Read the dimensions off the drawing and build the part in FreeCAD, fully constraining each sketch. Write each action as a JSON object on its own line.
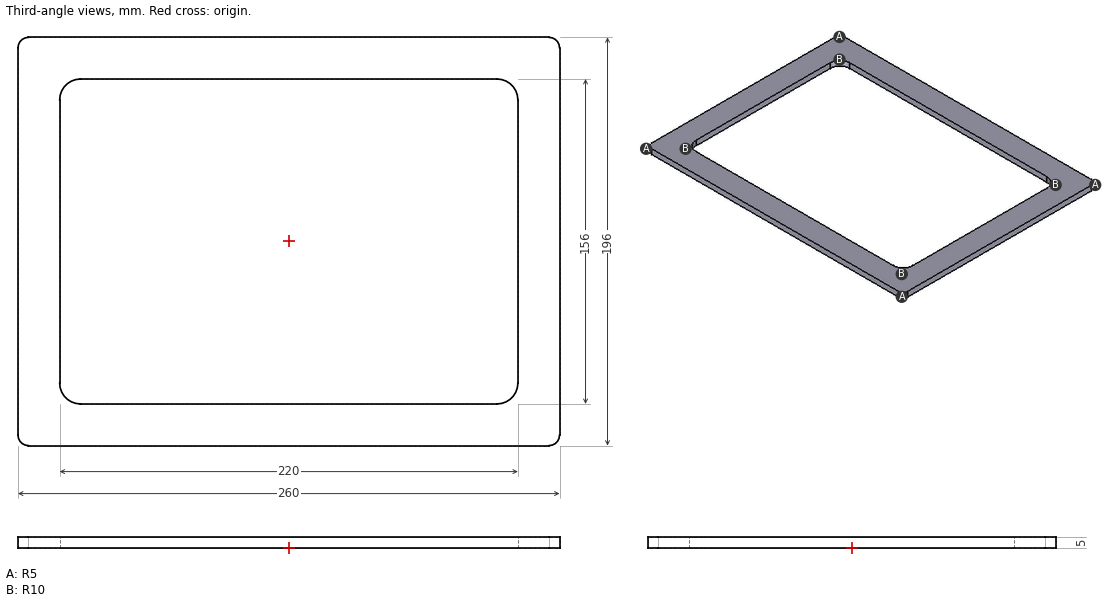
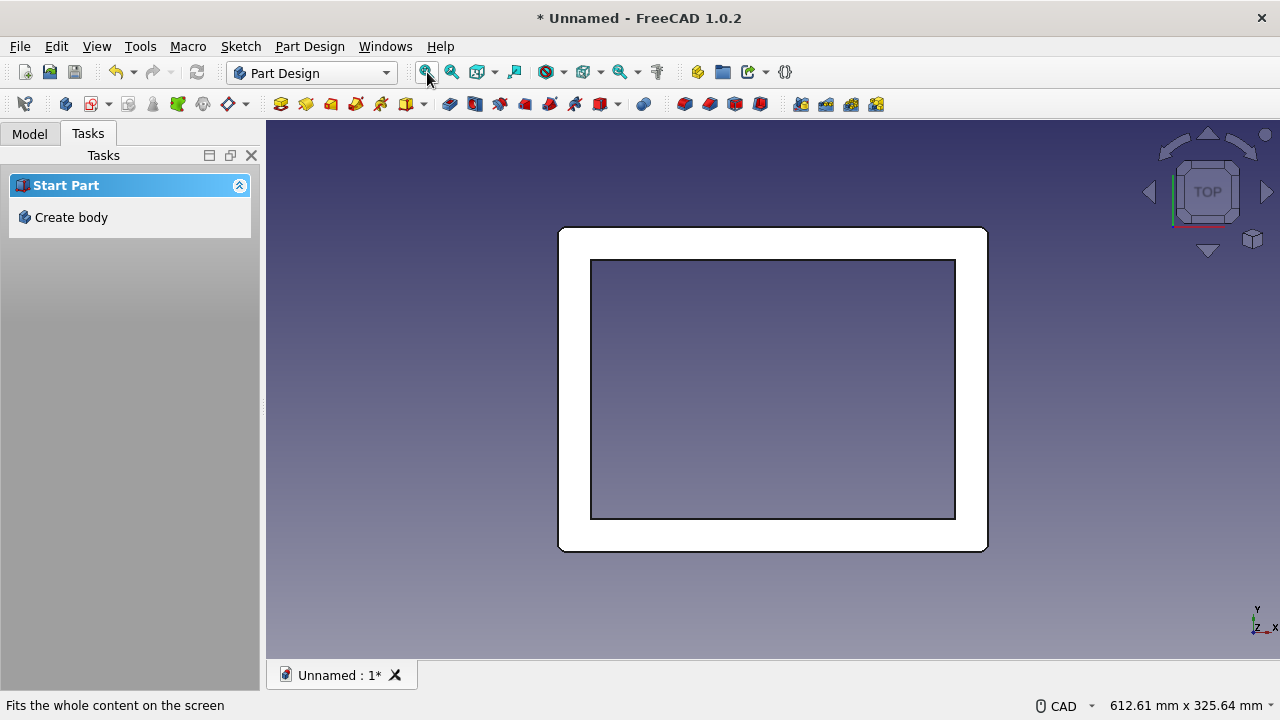
{"action": "key", "text": "0"}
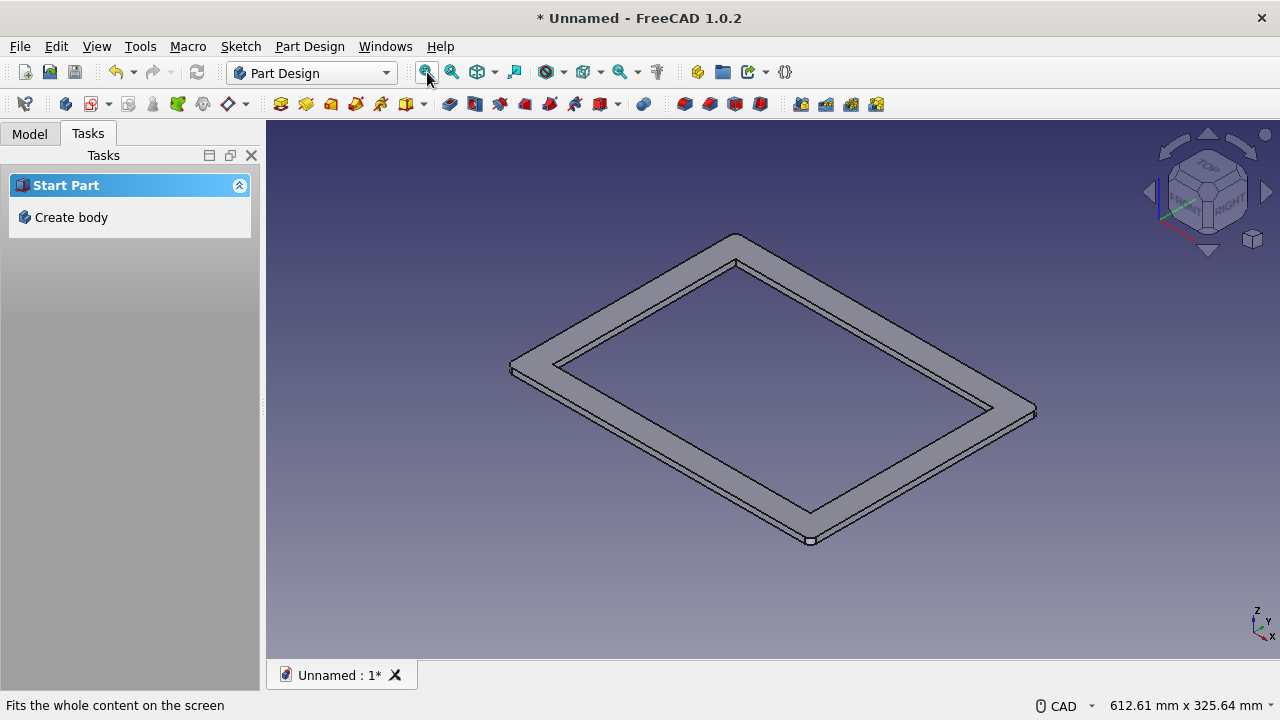
{"action": "scroll", "coordinate": [736, 261], "scroll_direction": "up", "scroll_amount": 8}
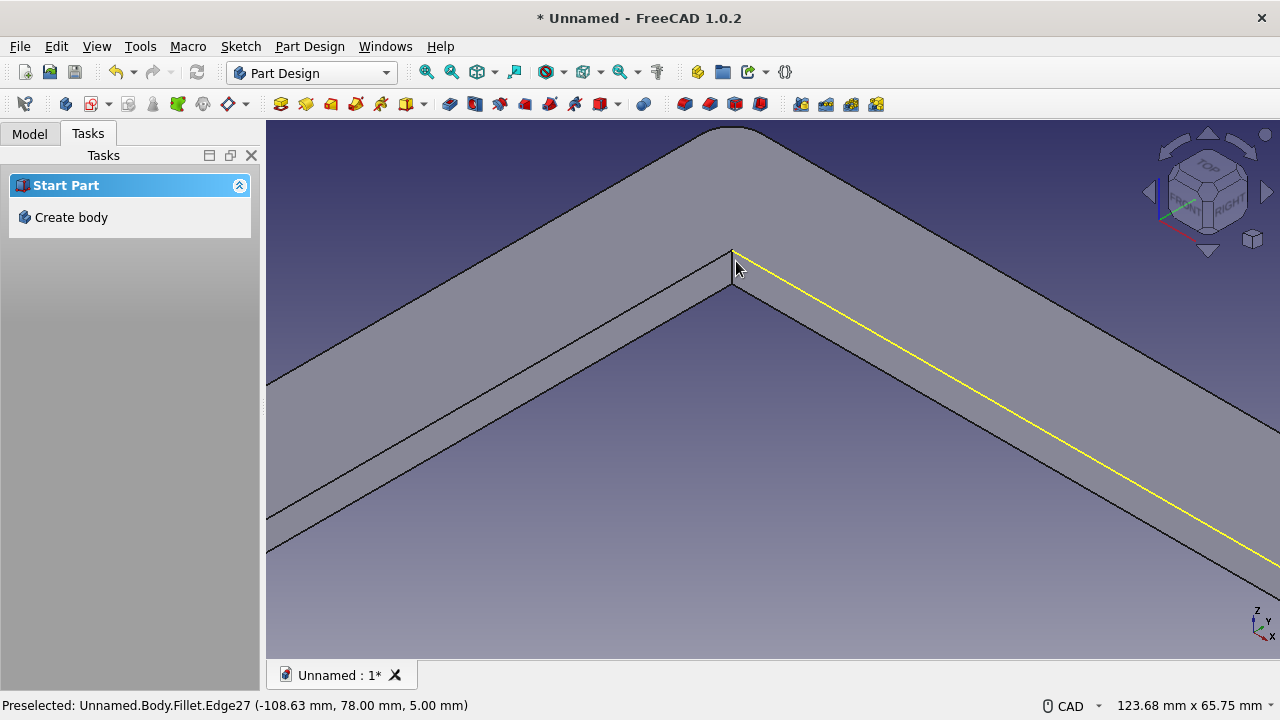
{"action": "left_click", "coordinate": [427, 72]}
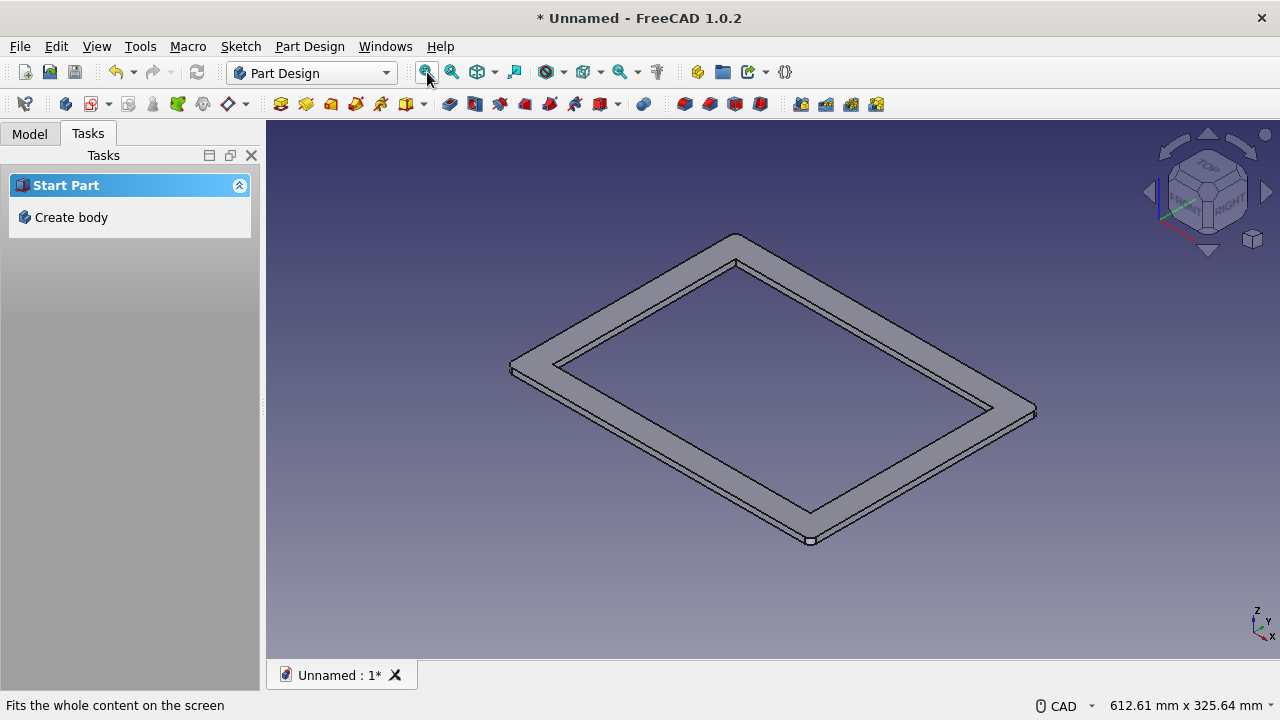
{"action": "key", "text": "1"}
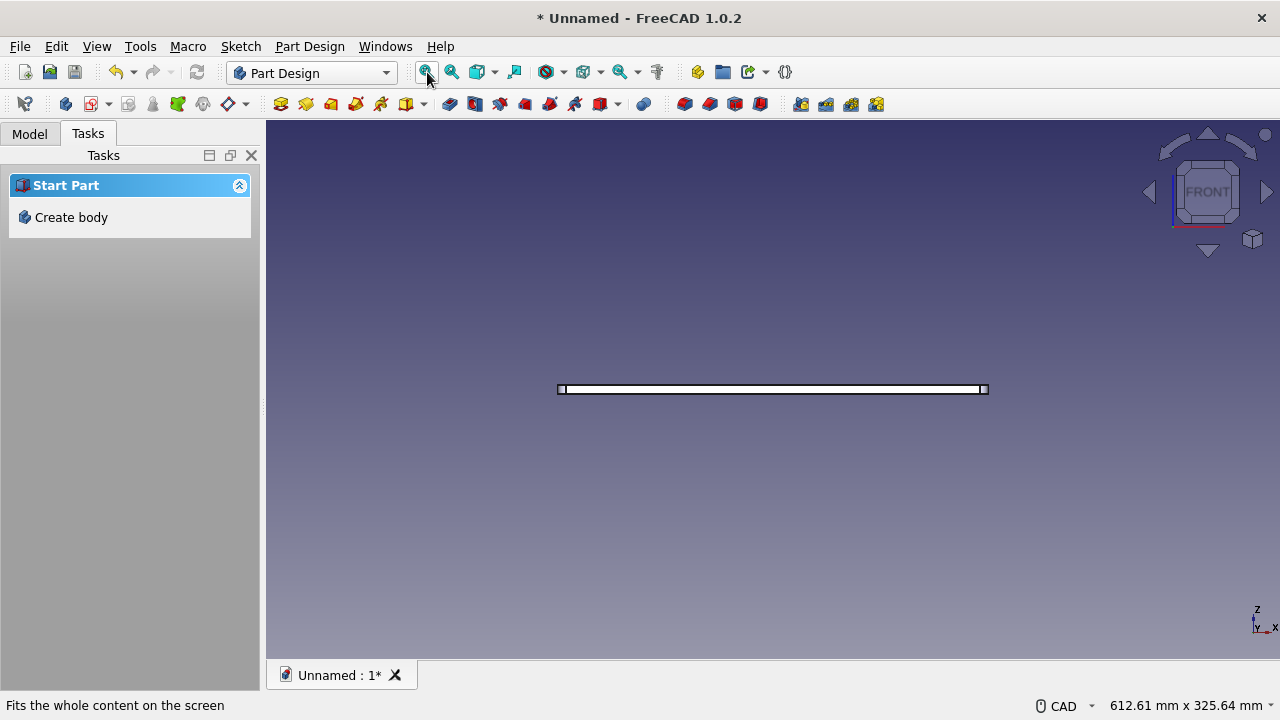
{"action": "left_click", "coordinate": [427, 72]}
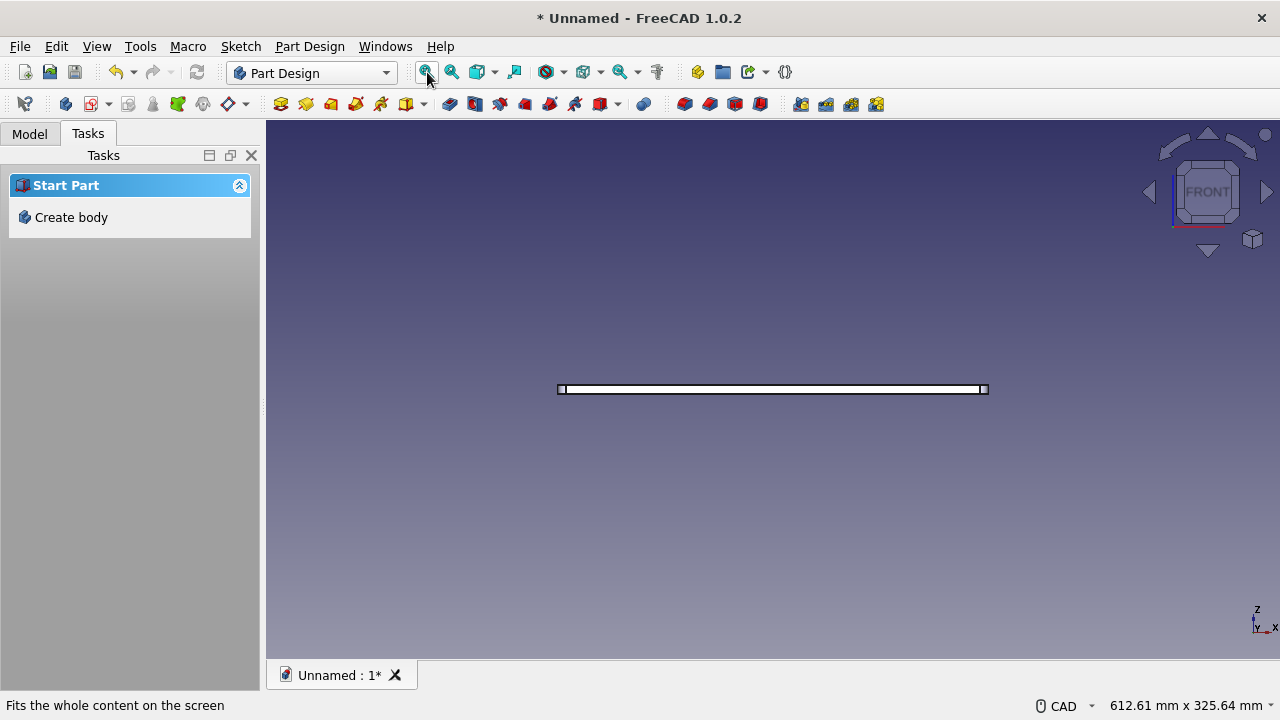
{"action": "scroll", "coordinate": [591, 389], "scroll_direction": "up", "scroll_amount": 8}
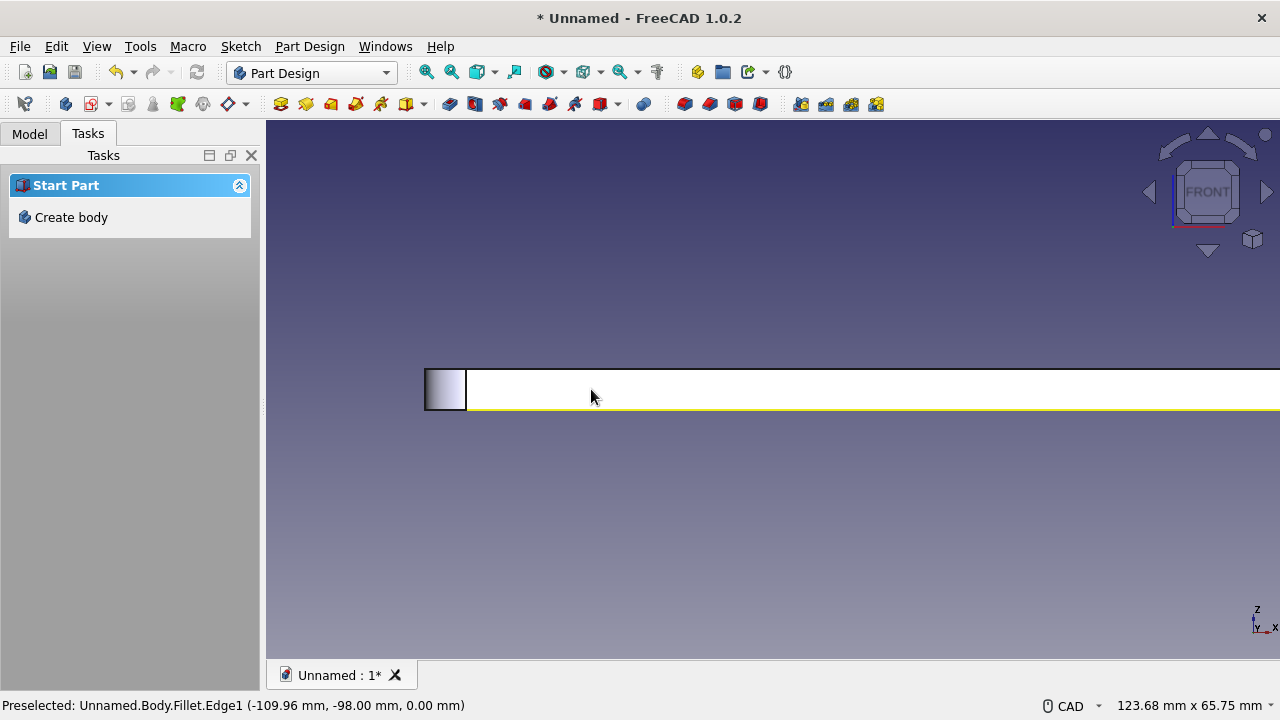
{"action": "left_click", "coordinate": [427, 72]}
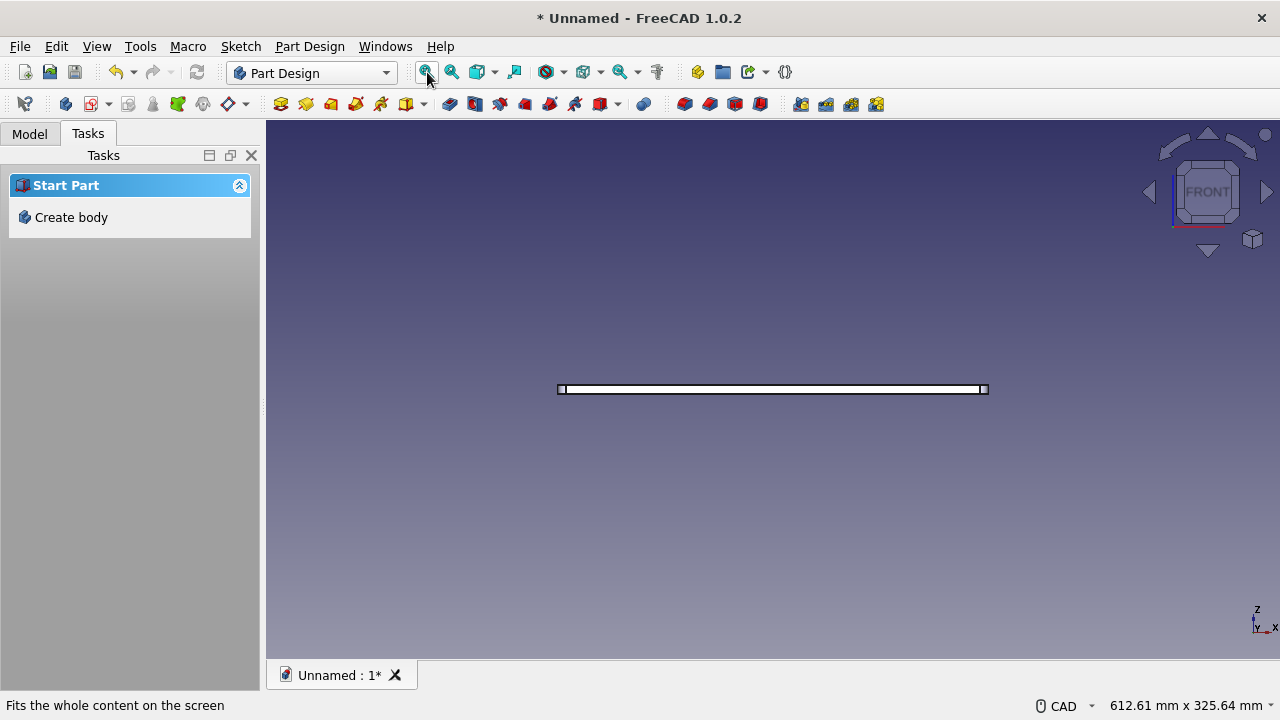
{"action": "key", "text": "3"}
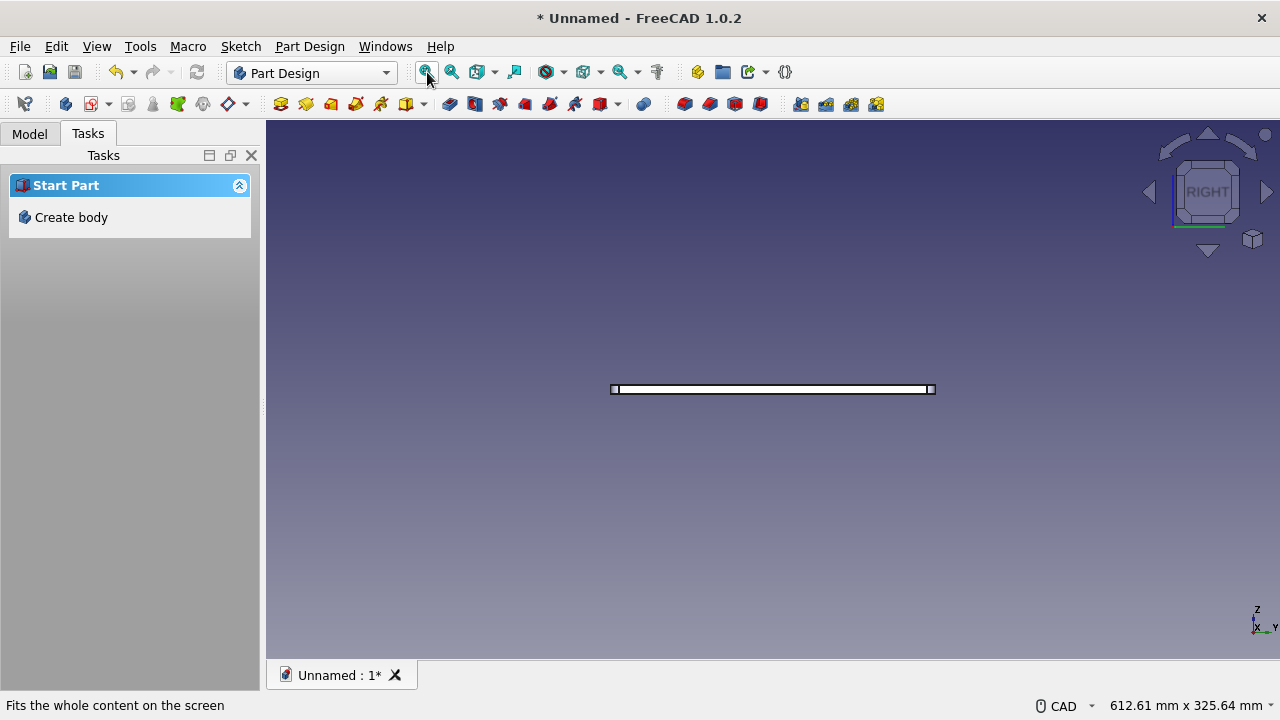
{"action": "left_click", "coordinate": [427, 72]}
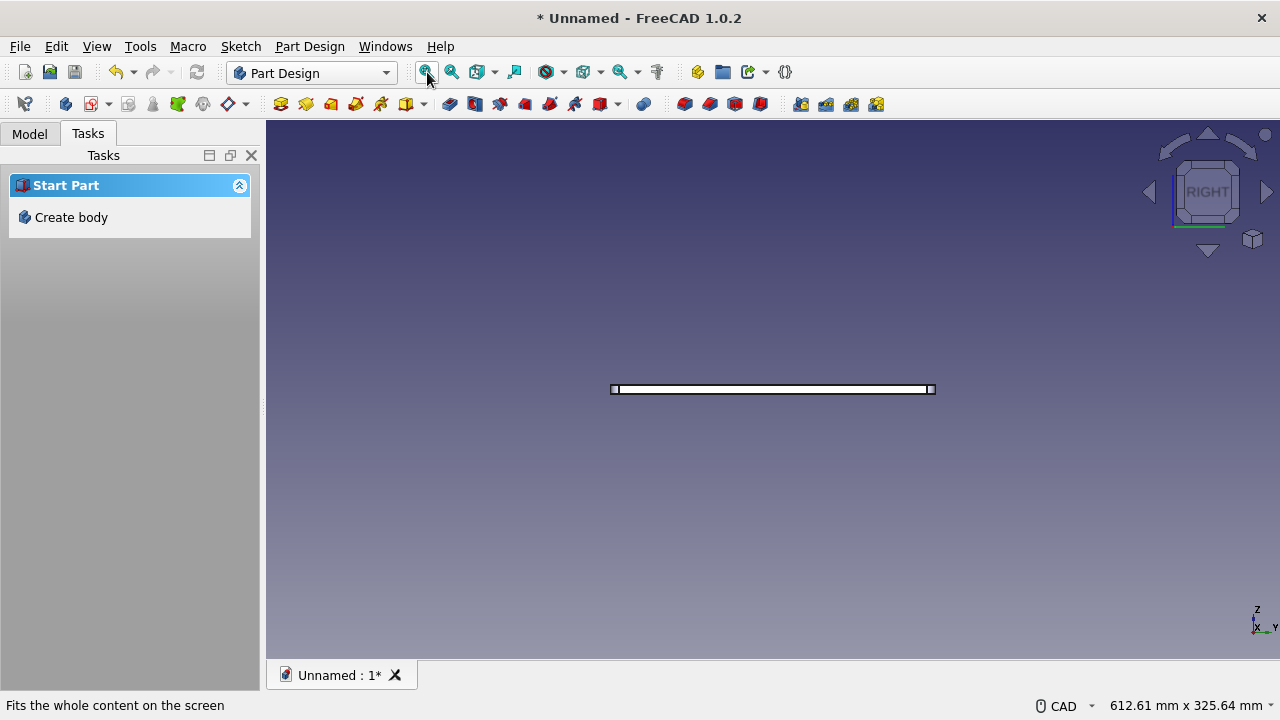
{"action": "scroll", "coordinate": [902, 388], "scroll_direction": "up", "scroll_amount": 8}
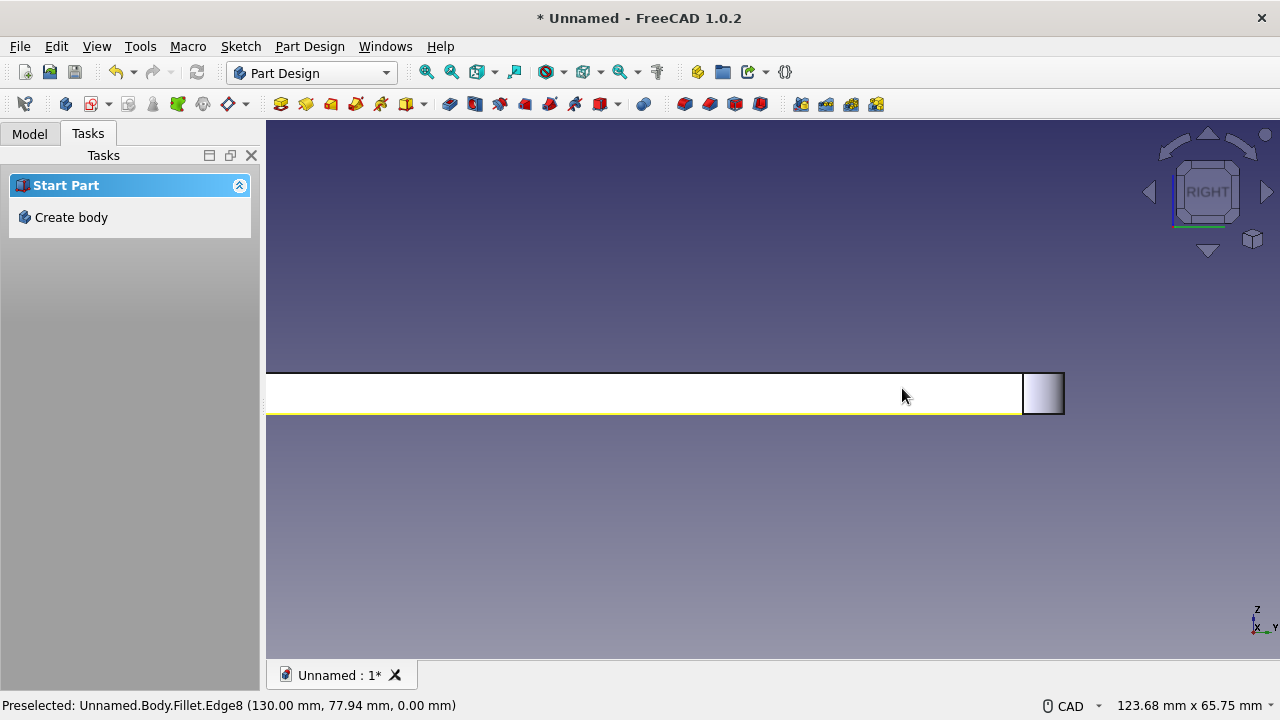
{"action": "left_click", "coordinate": [427, 72]}